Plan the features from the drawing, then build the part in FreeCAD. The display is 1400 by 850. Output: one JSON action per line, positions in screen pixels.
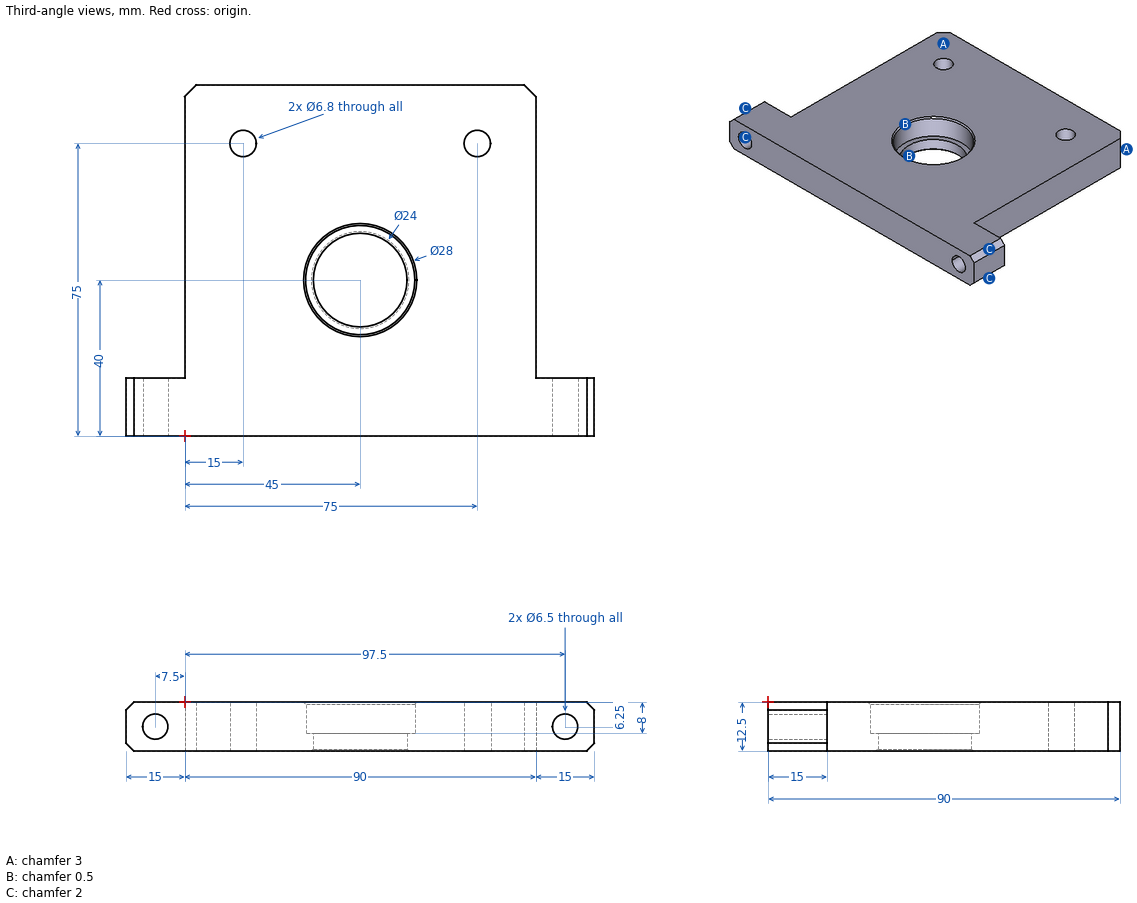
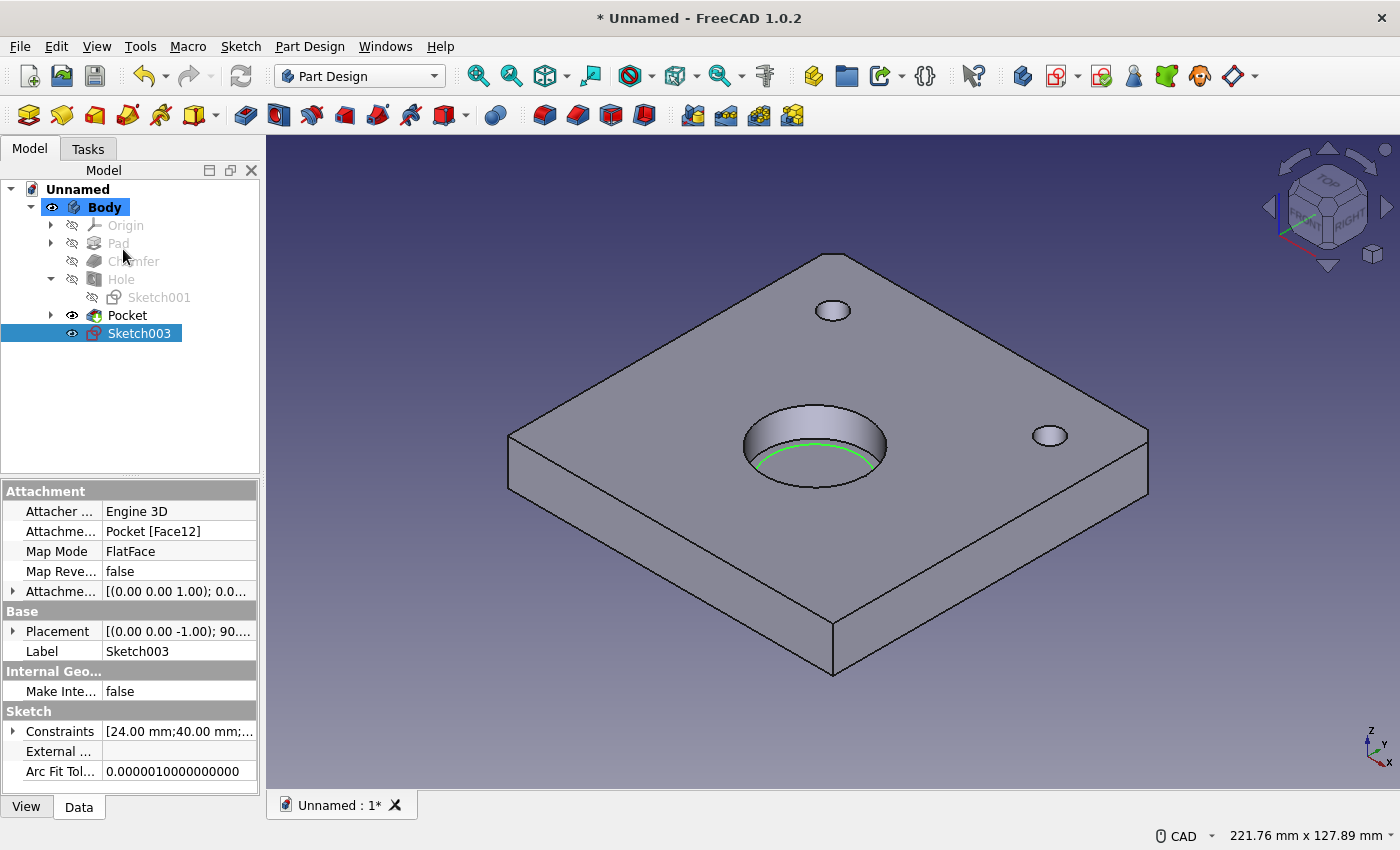
{"action": "left_click", "coordinate": [246, 116]}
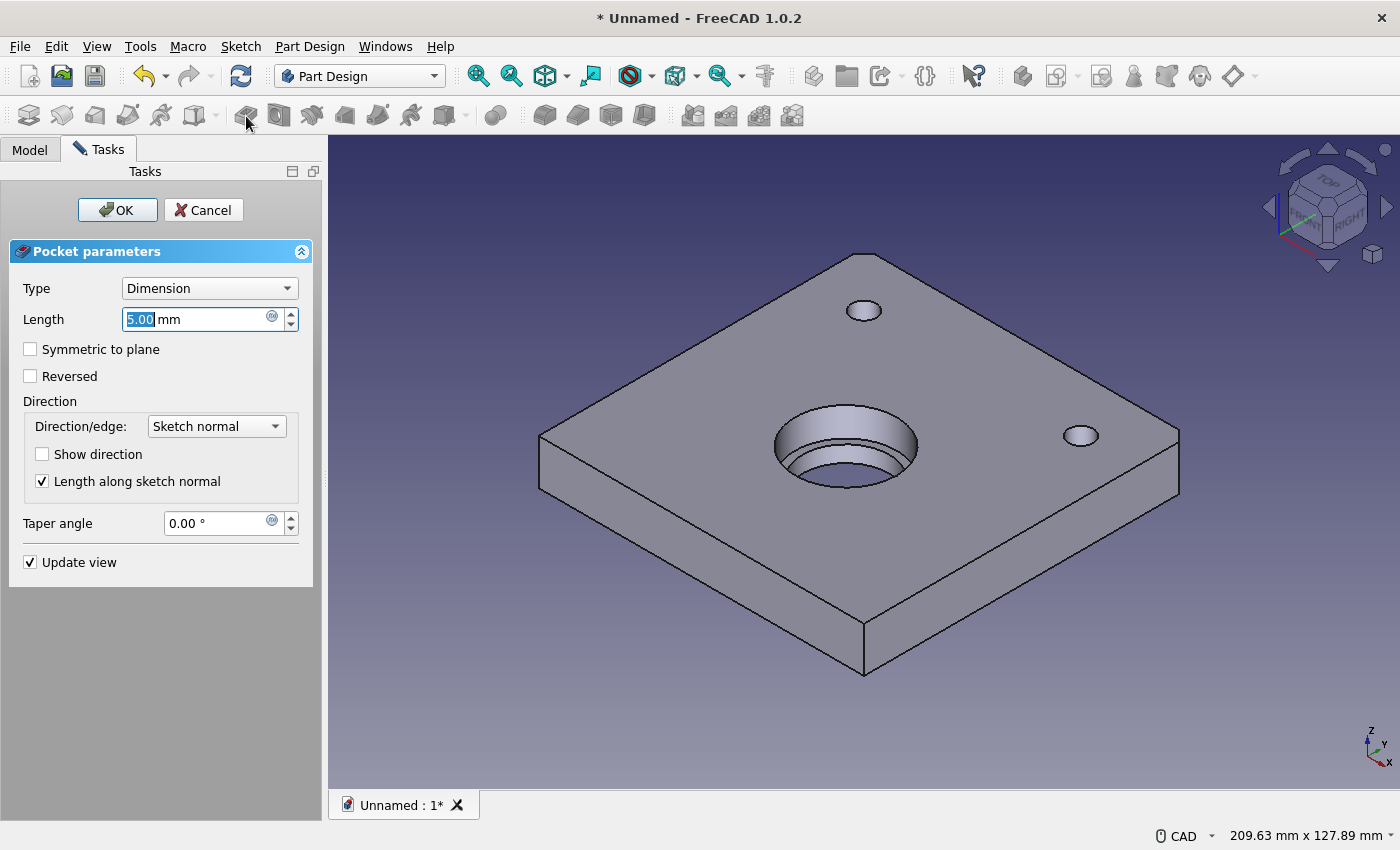
{"action": "left_click", "coordinate": [210, 288]}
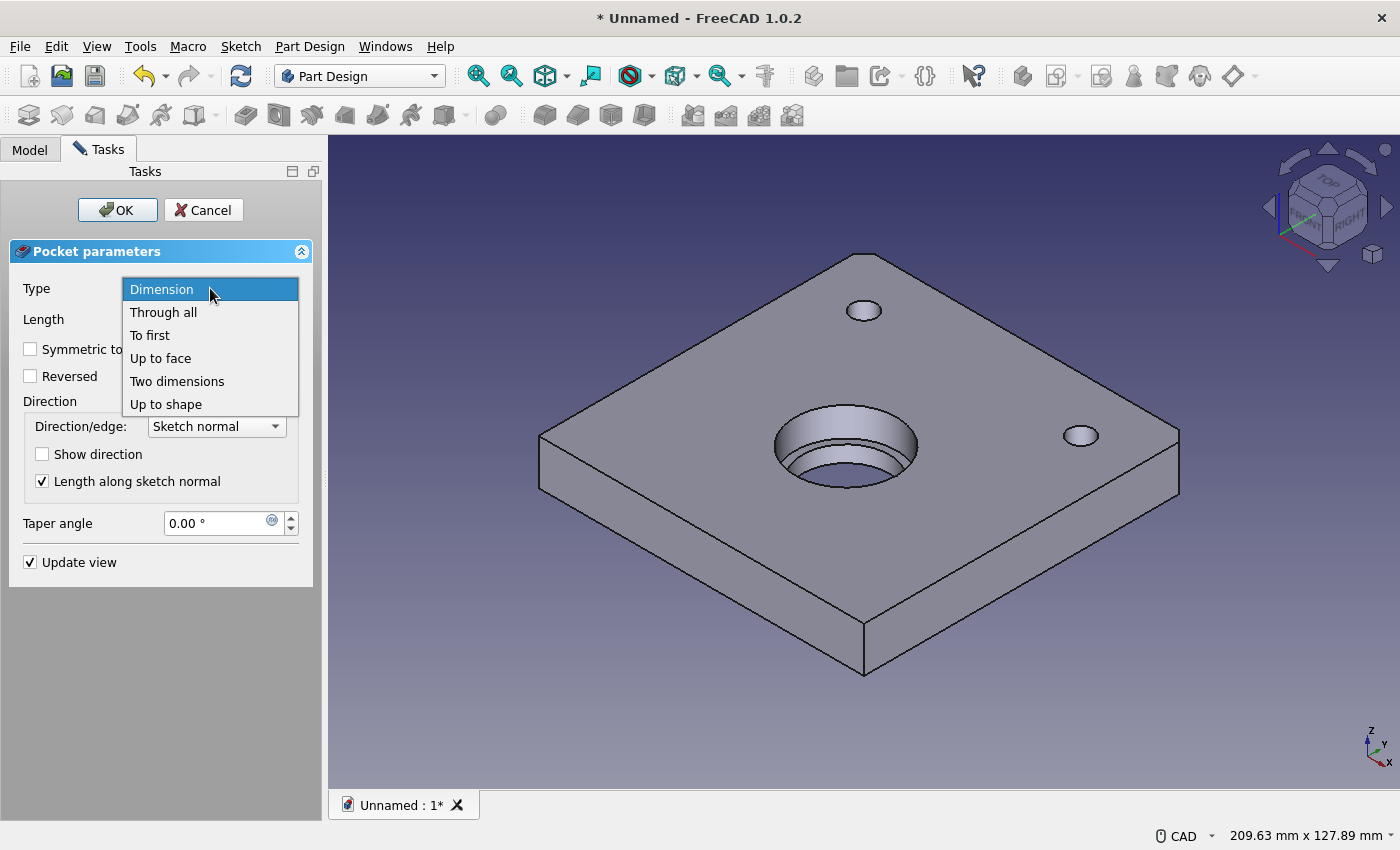
{"action": "left_click", "coordinate": [208, 312]}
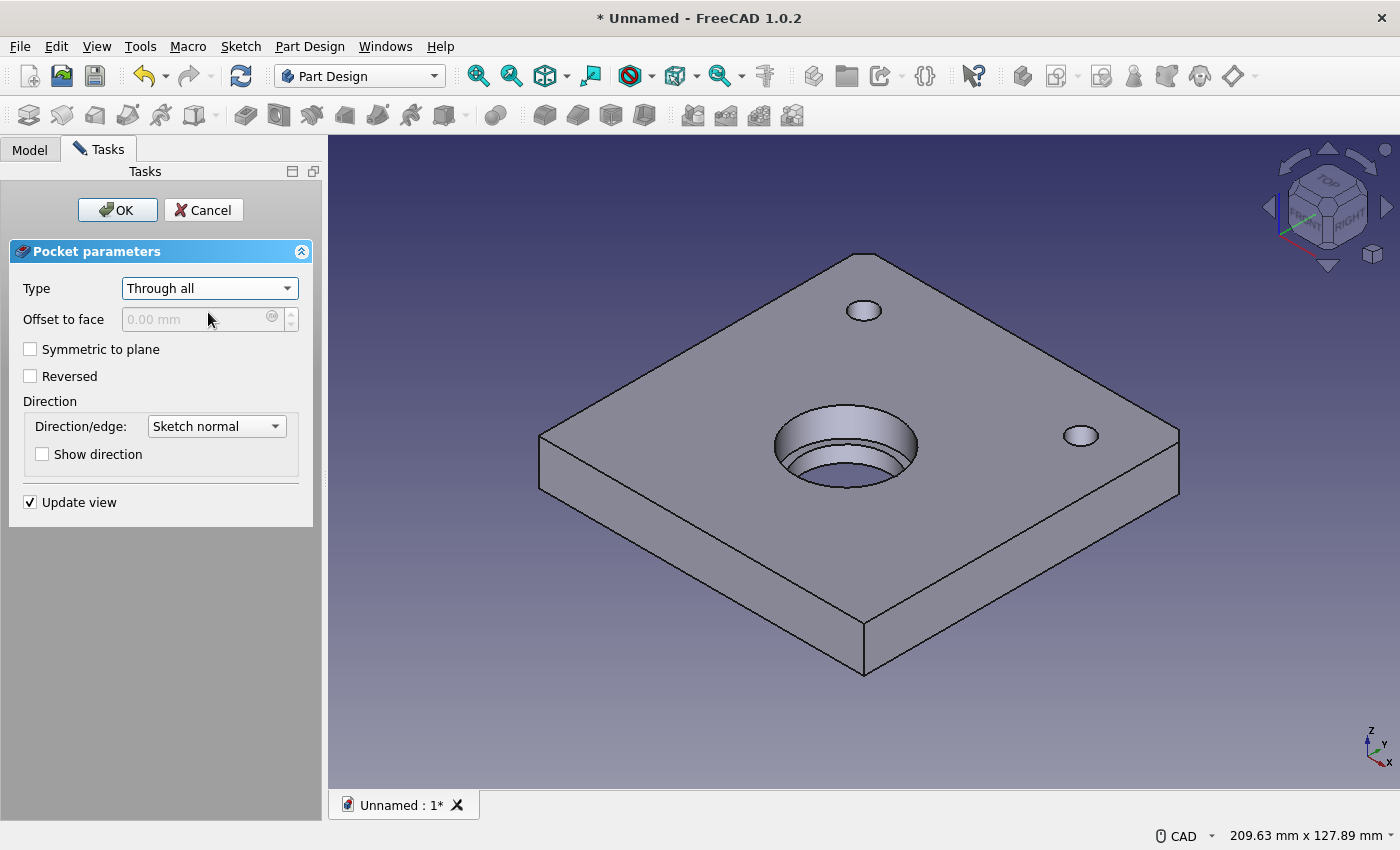
{"action": "left_click", "coordinate": [118, 210]}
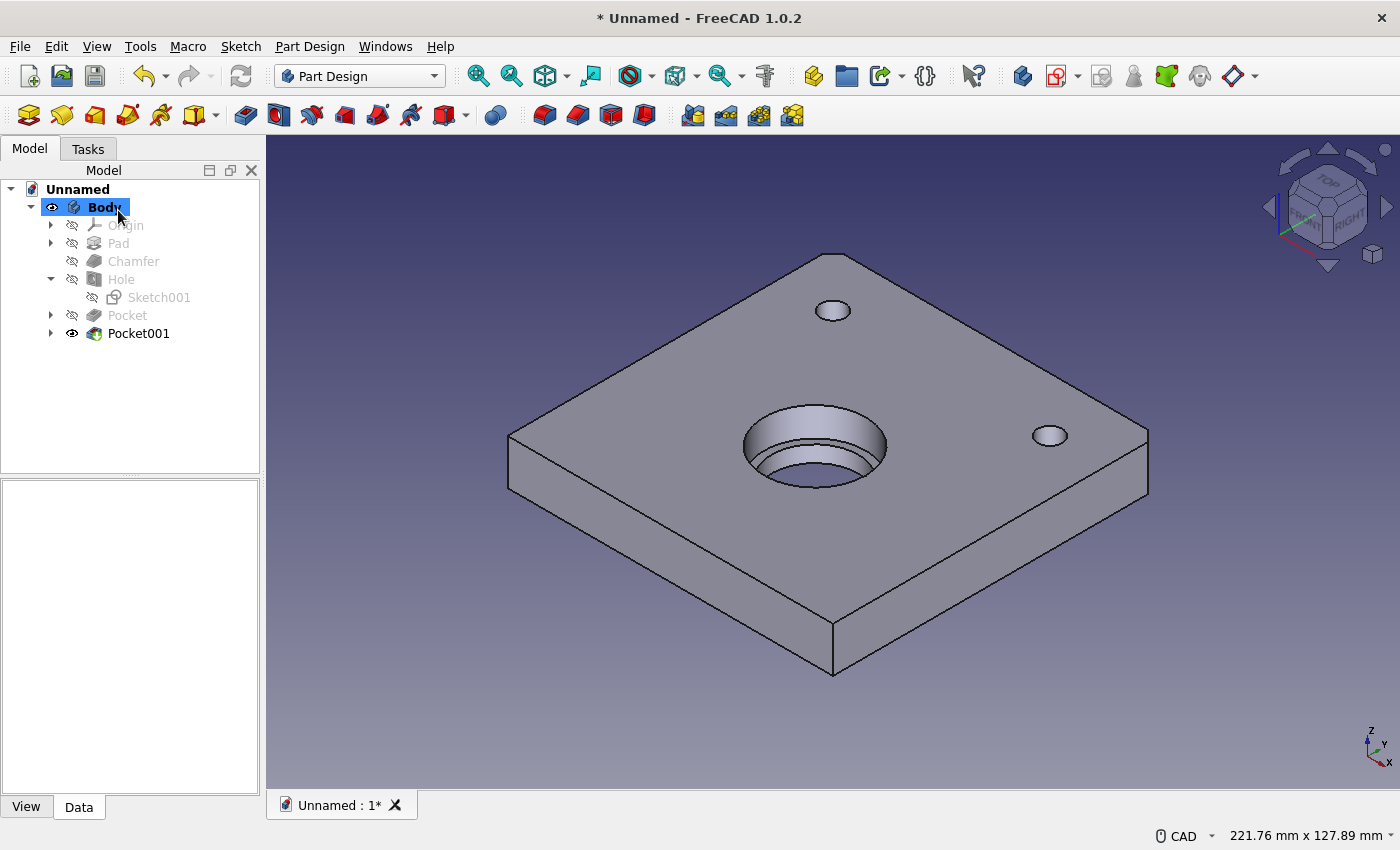
{"action": "left_click", "coordinate": [764, 416]}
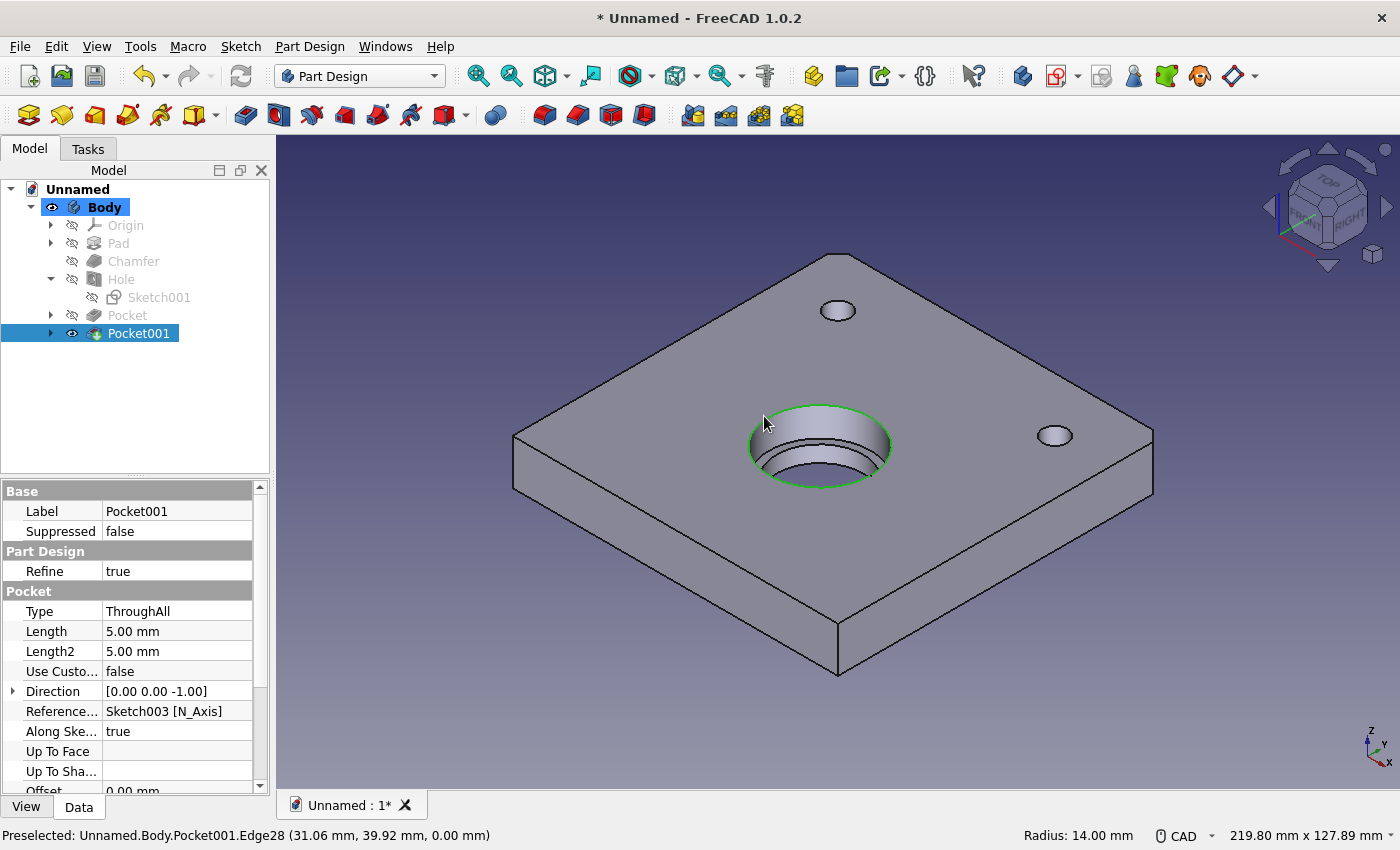
{"action": "key", "text": "2"}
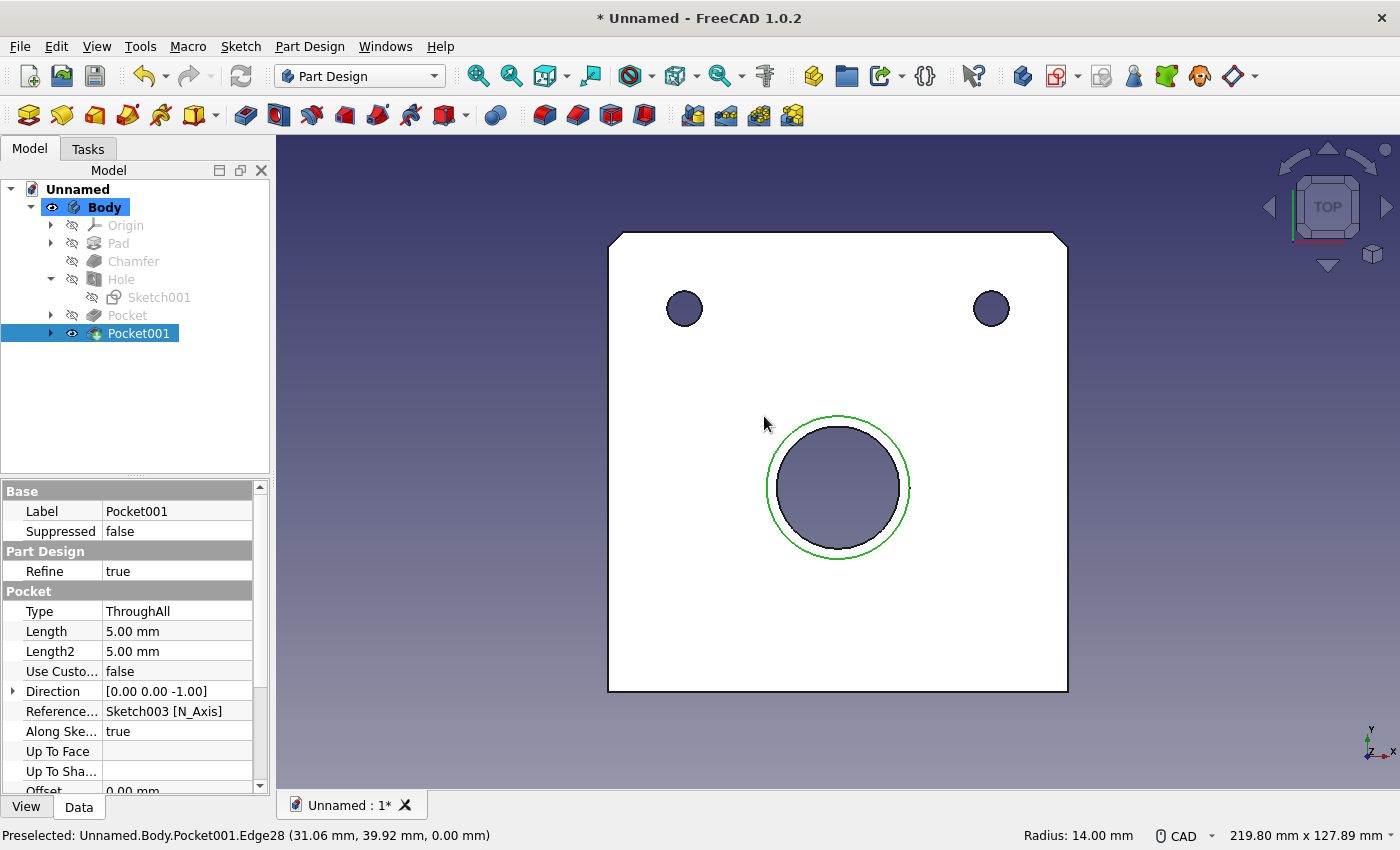
{"action": "key", "text": "0"}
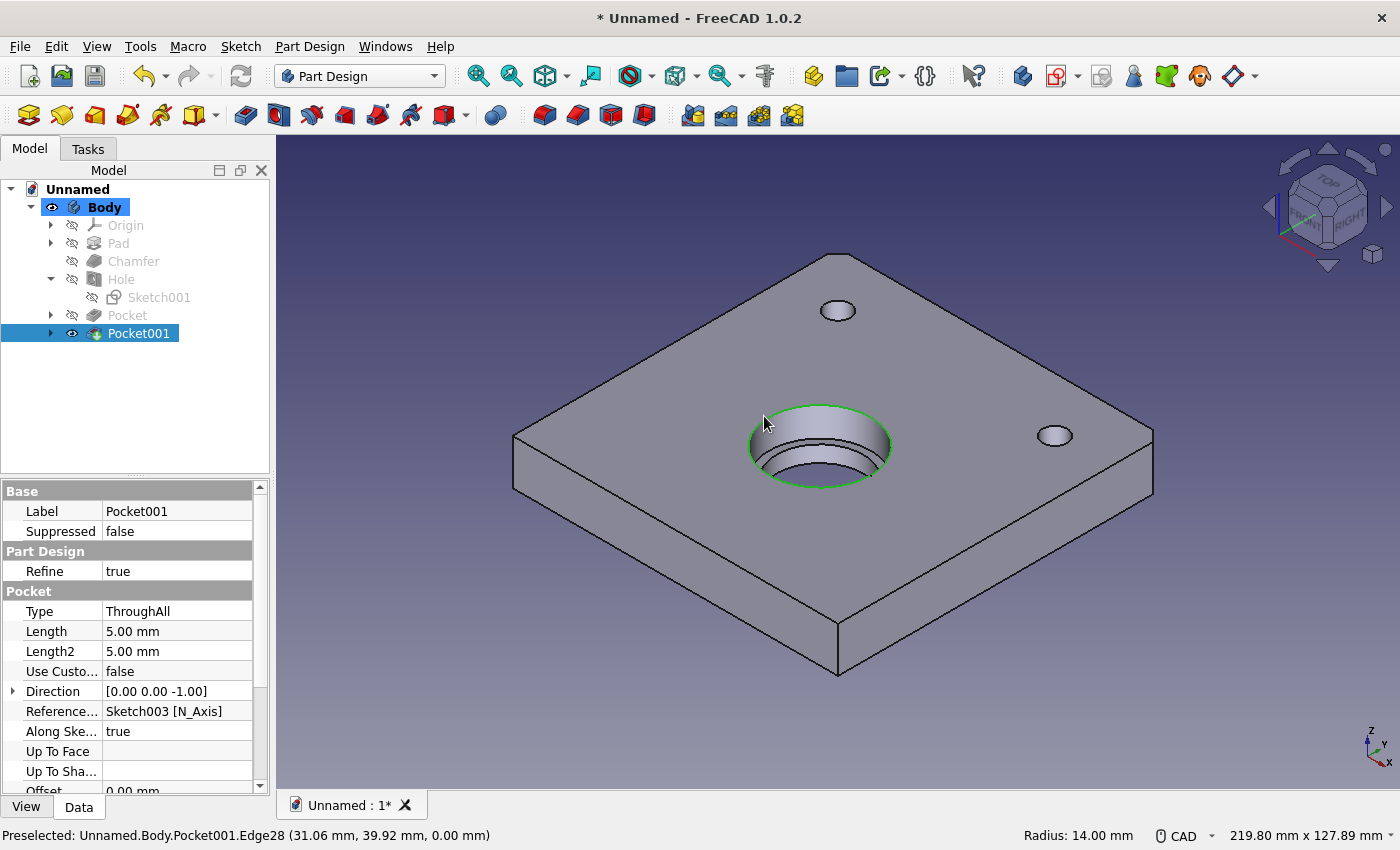
{"action": "key", "text": "1"}